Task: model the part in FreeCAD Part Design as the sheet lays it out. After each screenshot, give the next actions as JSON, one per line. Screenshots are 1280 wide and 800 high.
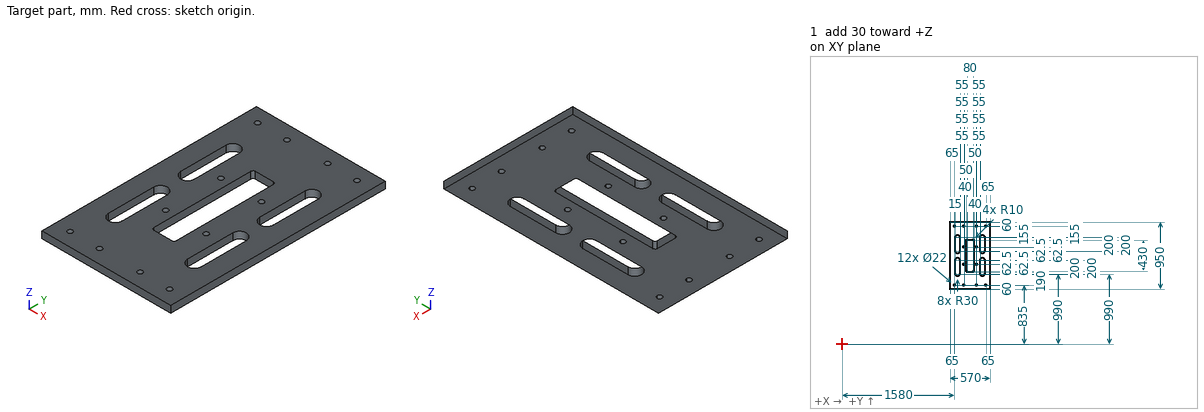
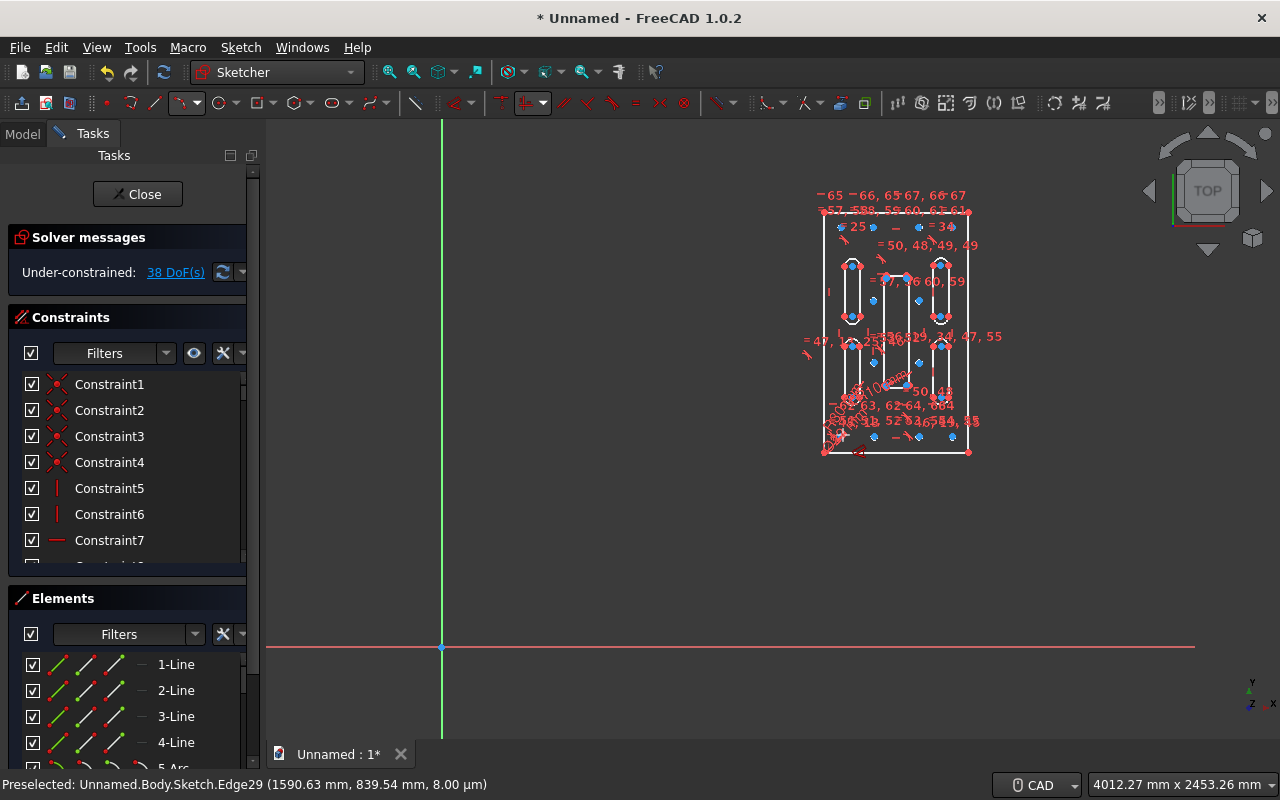
{"action": "scroll", "coordinate": [901, 388], "scroll_direction": "up", "scroll_amount": 5}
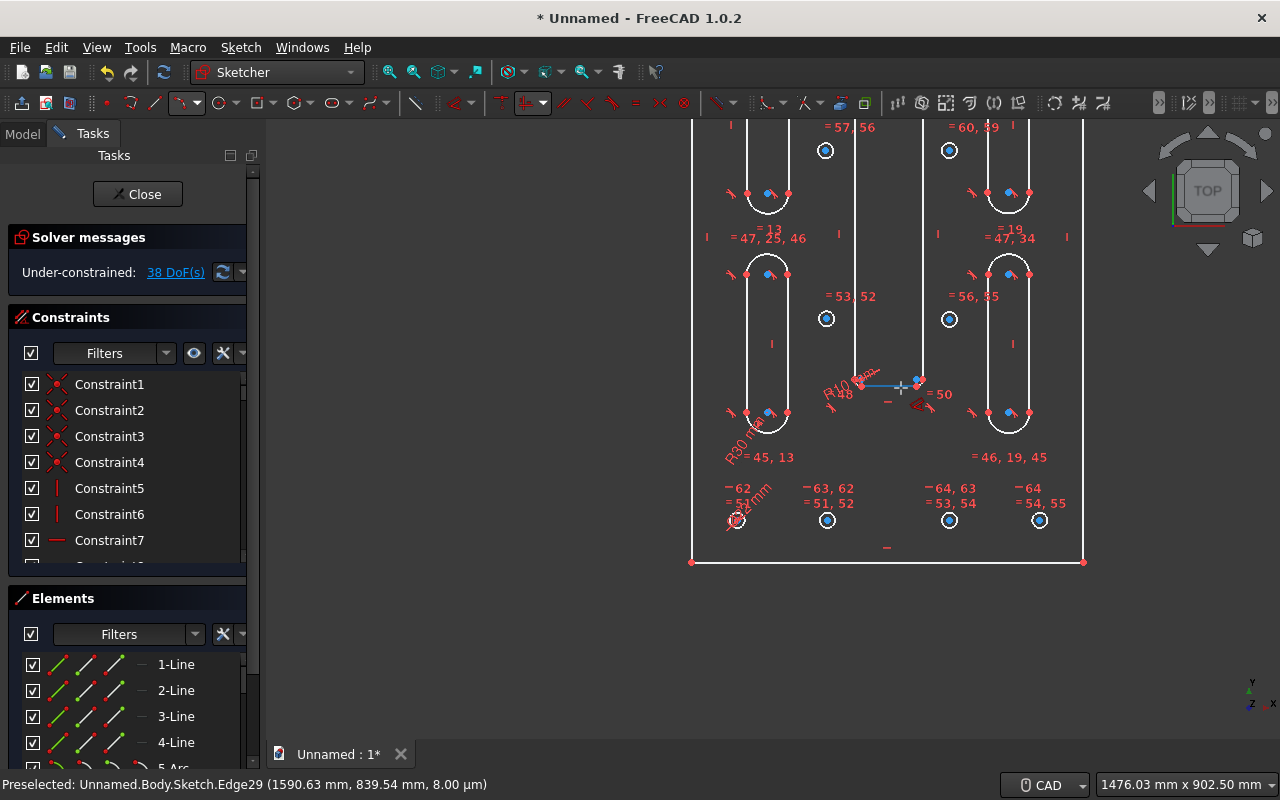
{"action": "left_click", "coordinate": [900, 386]}
{"action": "left_click", "coordinate": [889, 352]}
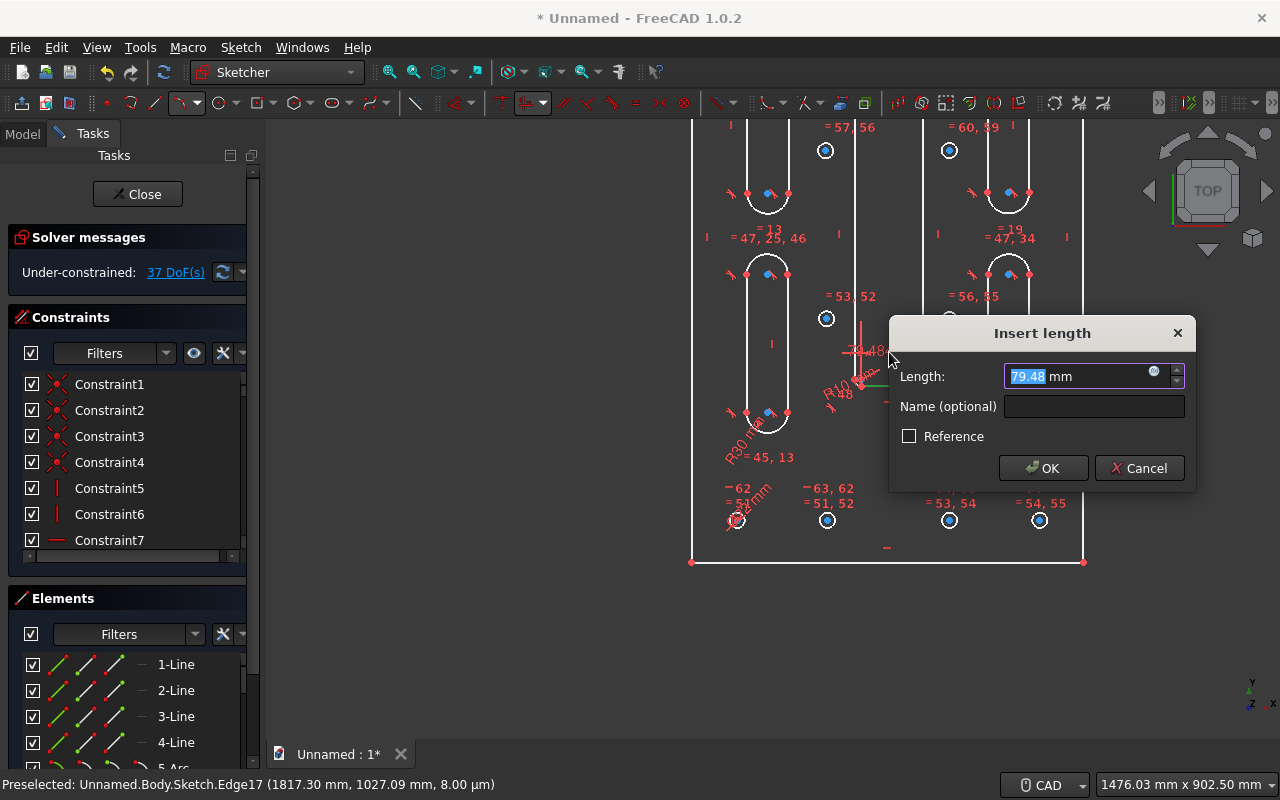
{"action": "type", "text": "80"}
{"action": "key", "text": "Return"}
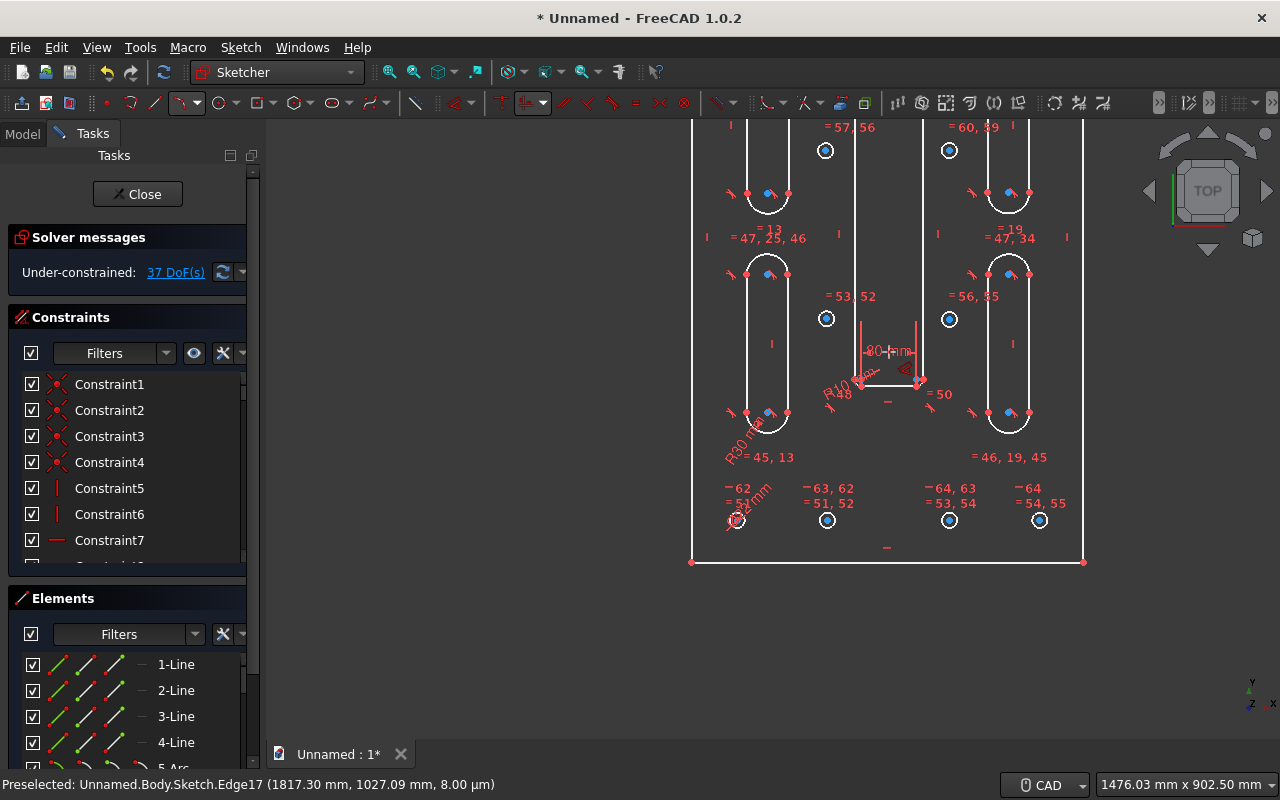
{"action": "left_click", "coordinate": [692, 367]}
{"action": "left_click", "coordinate": [726, 355]}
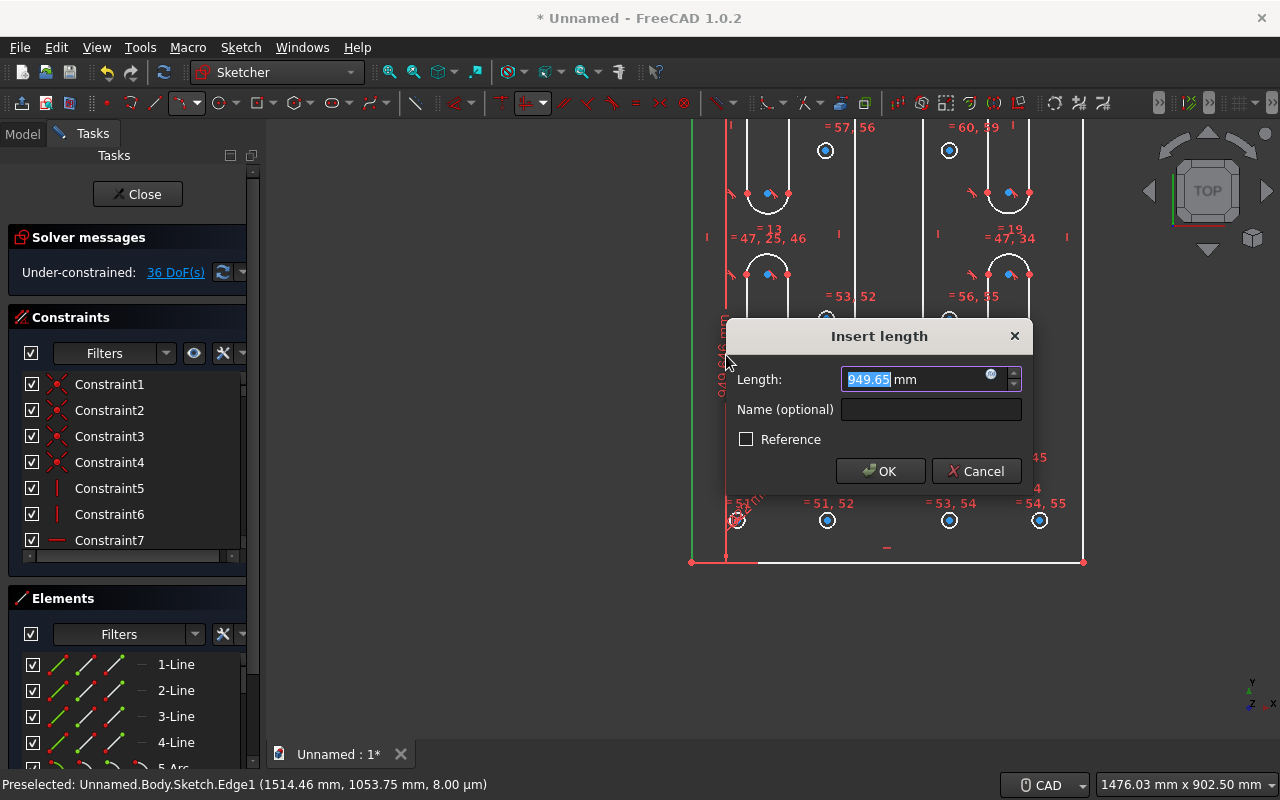
{"action": "type", "text": "950"}
{"action": "key", "text": "Return"}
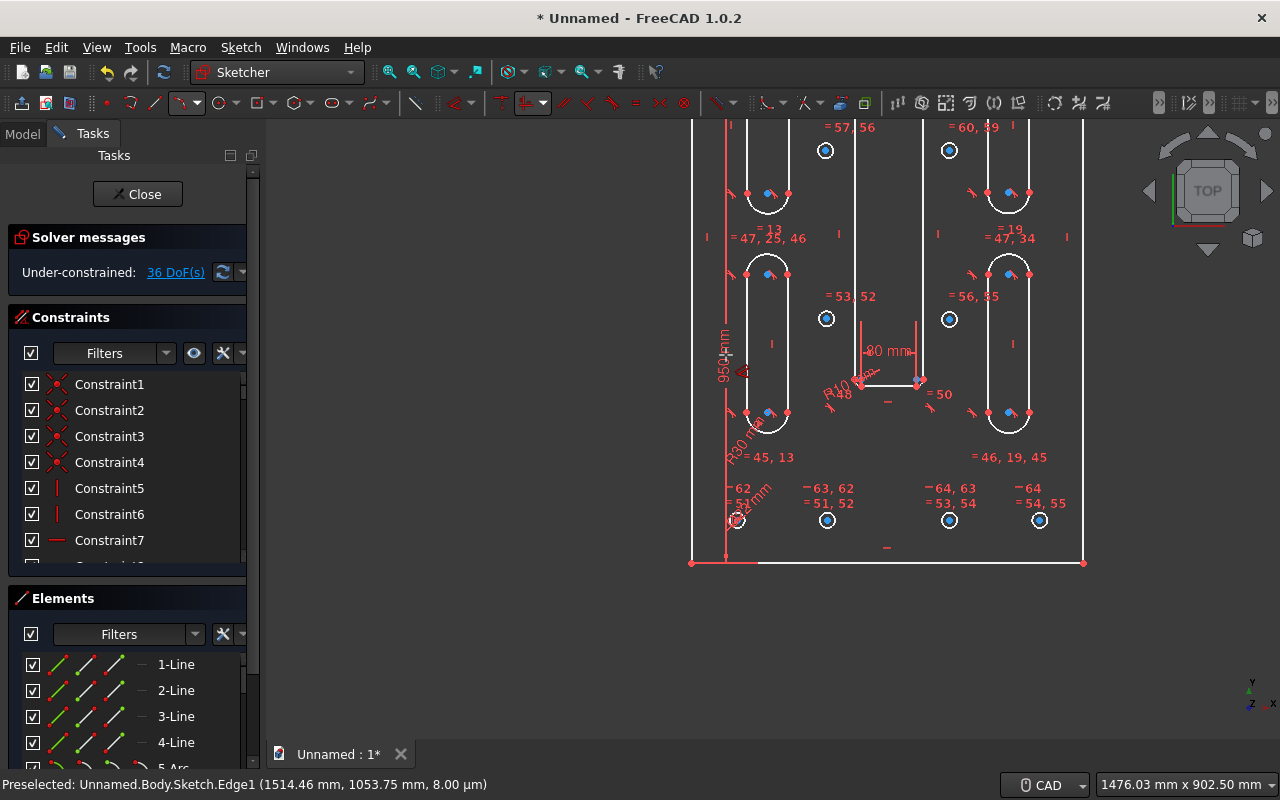
{"action": "left_click", "coordinate": [809, 563]}
{"action": "left_click", "coordinate": [888, 597]}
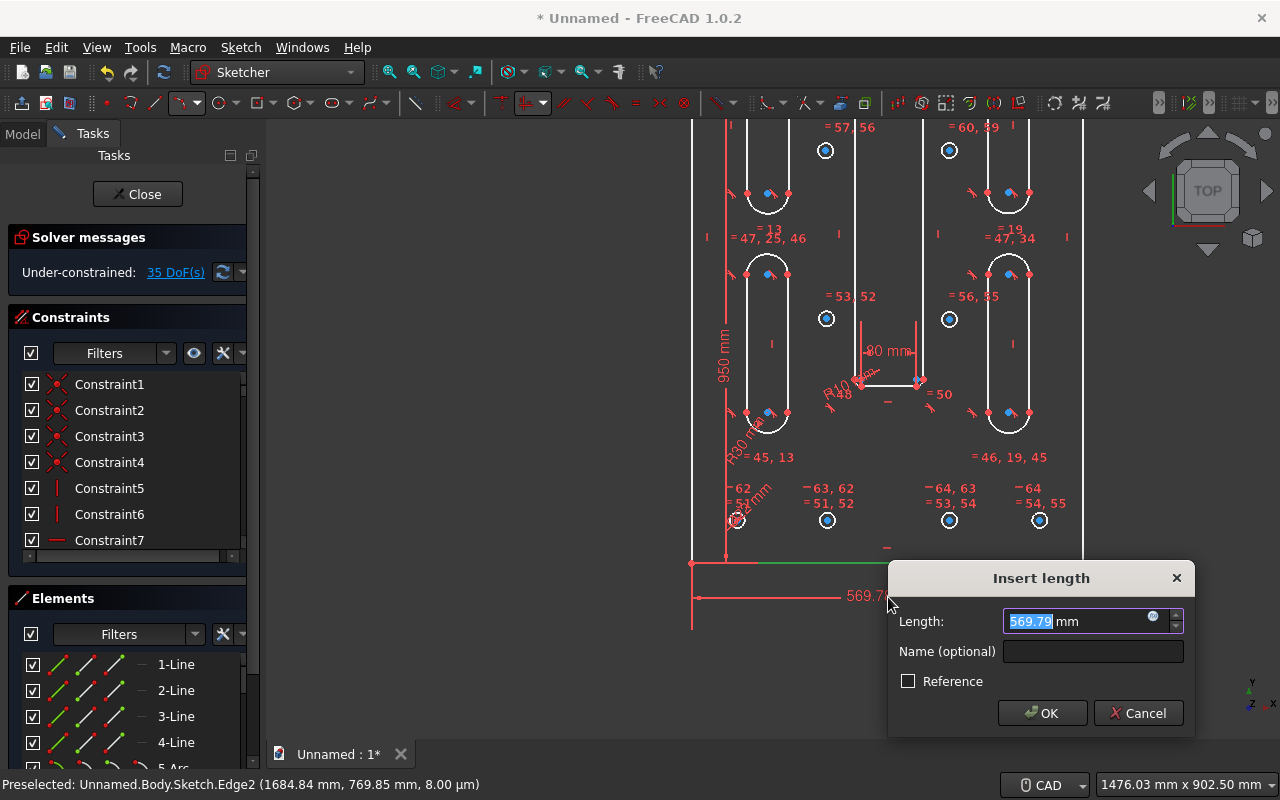
{"action": "type", "text": "570"}
{"action": "key", "text": "Return"}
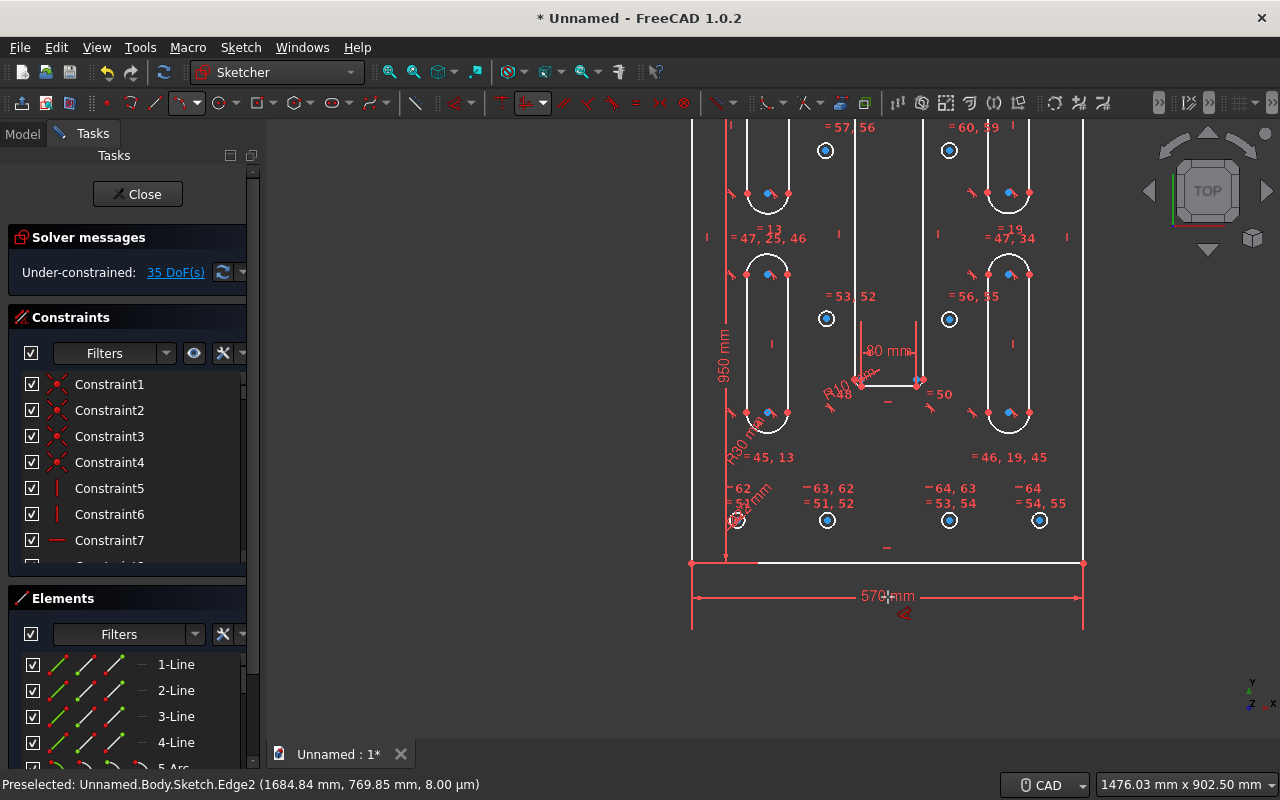
{"action": "left_click", "coordinate": [747, 371]}
{"action": "left_click", "coordinate": [713, 312]}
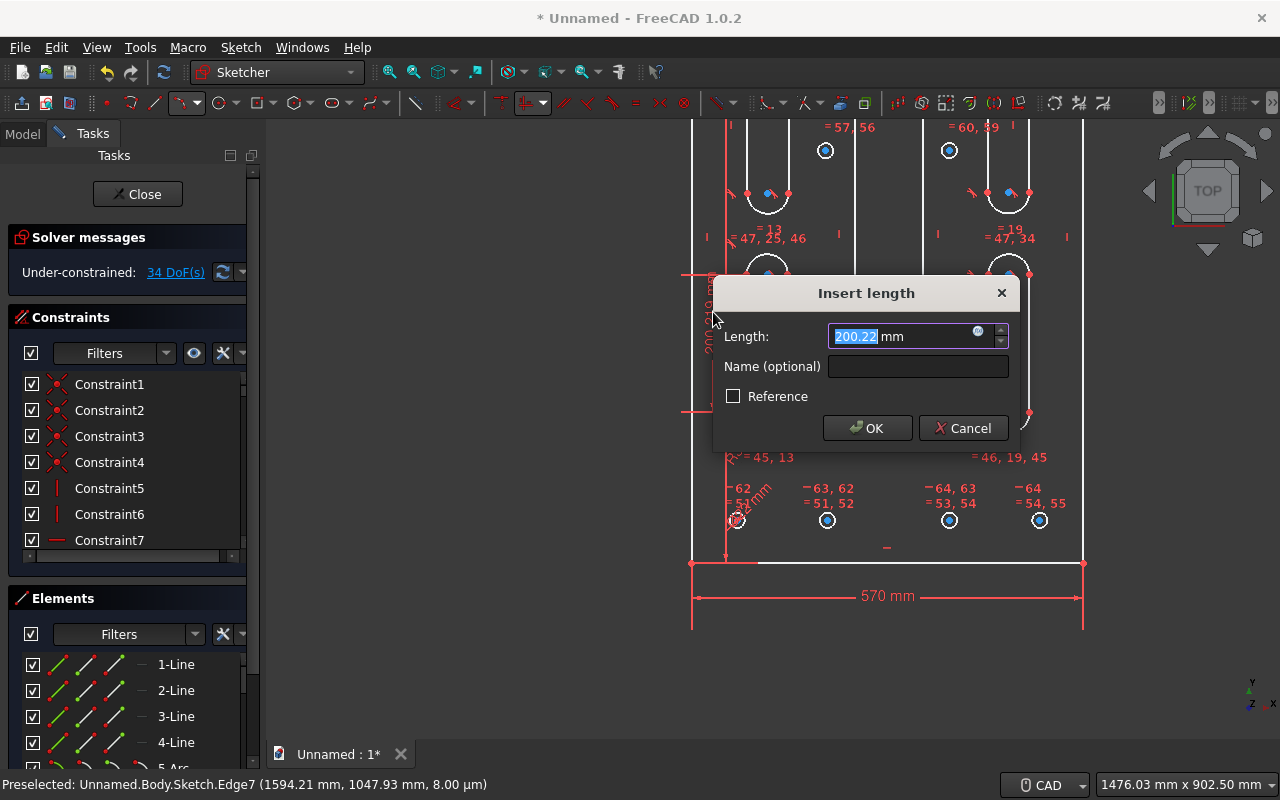
{"action": "type", "text": "200"}
{"action": "key", "text": "Return"}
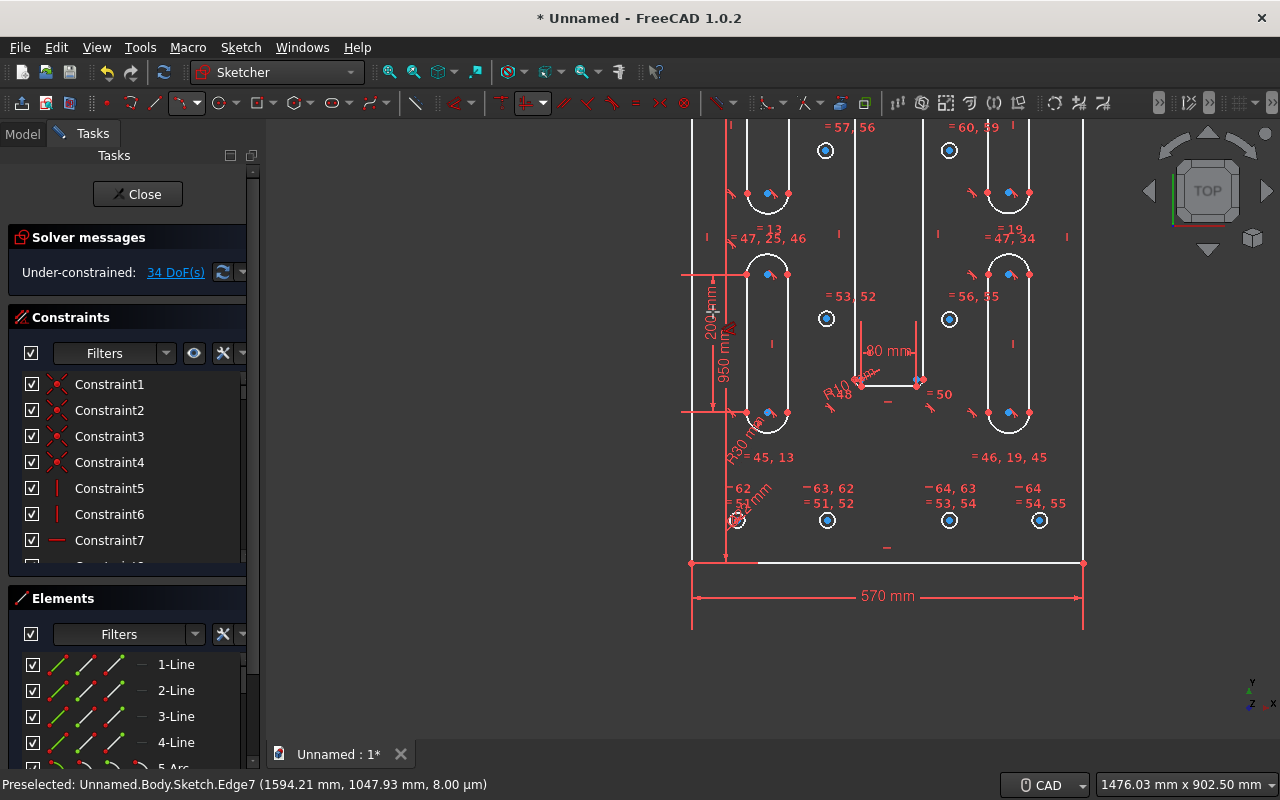
{"action": "left_click", "coordinate": [988, 371]}
{"action": "left_click", "coordinate": [954, 375]}